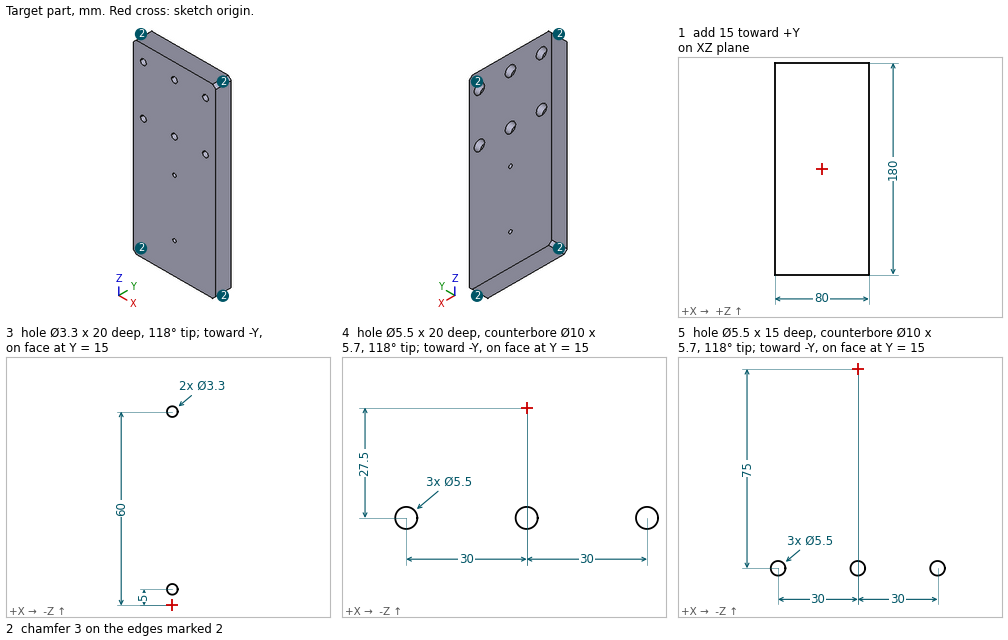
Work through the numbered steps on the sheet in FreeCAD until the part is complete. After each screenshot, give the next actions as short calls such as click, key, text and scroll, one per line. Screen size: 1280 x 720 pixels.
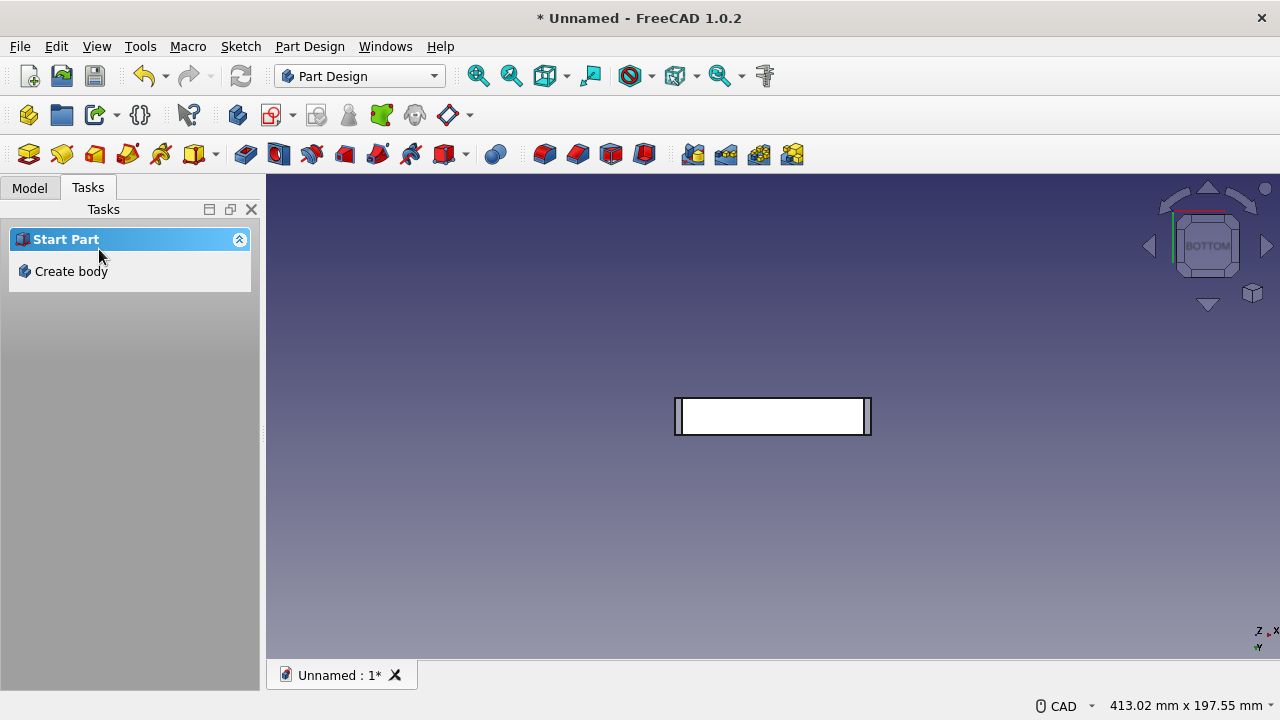
click(479, 76)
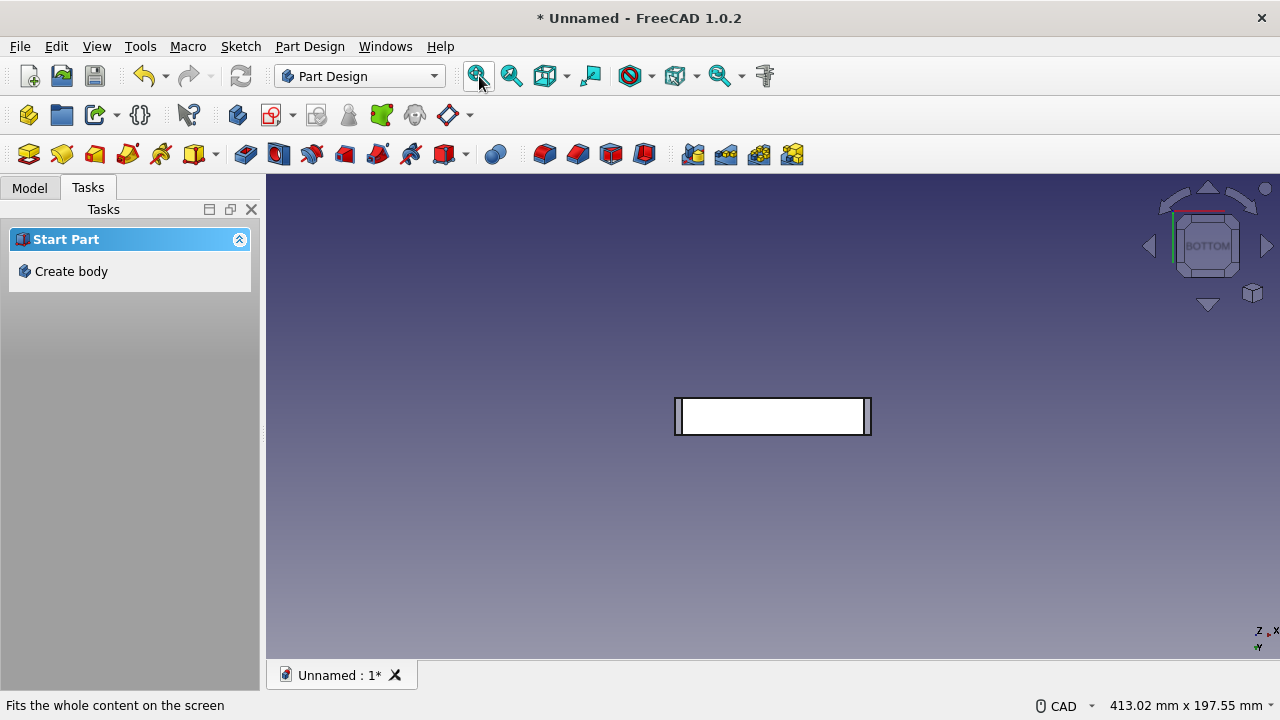
key(4)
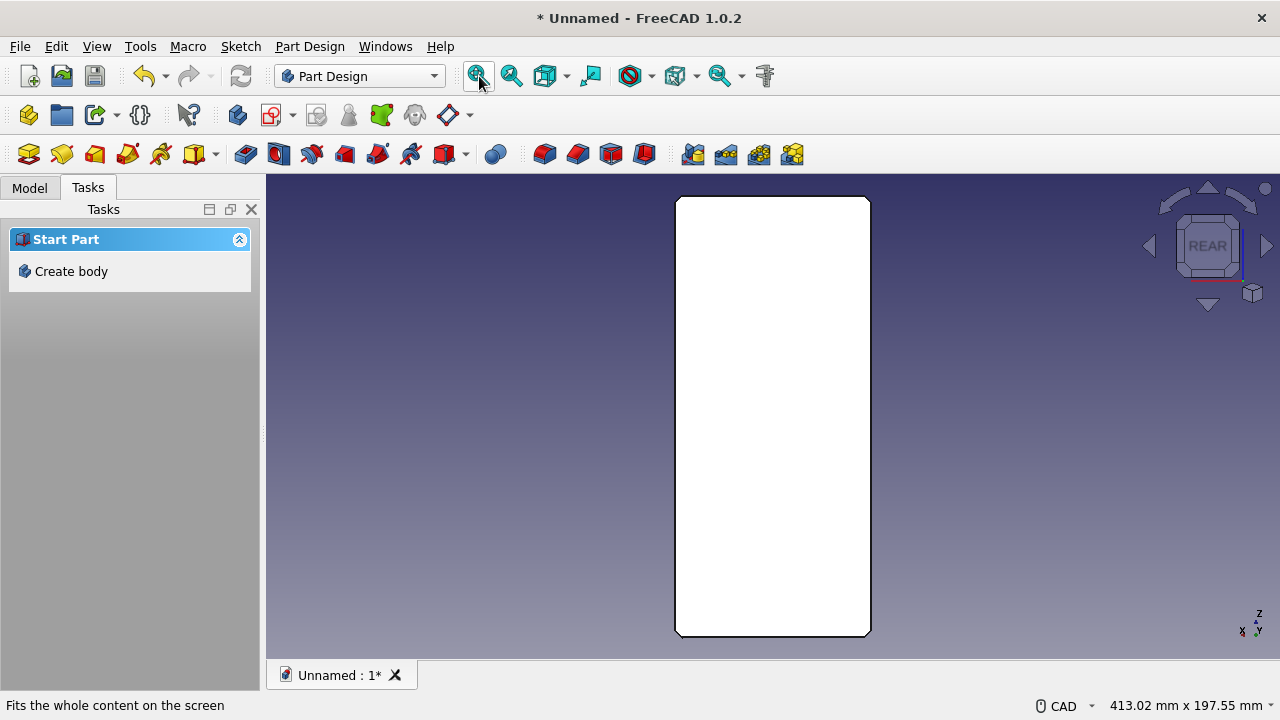
click(773, 352)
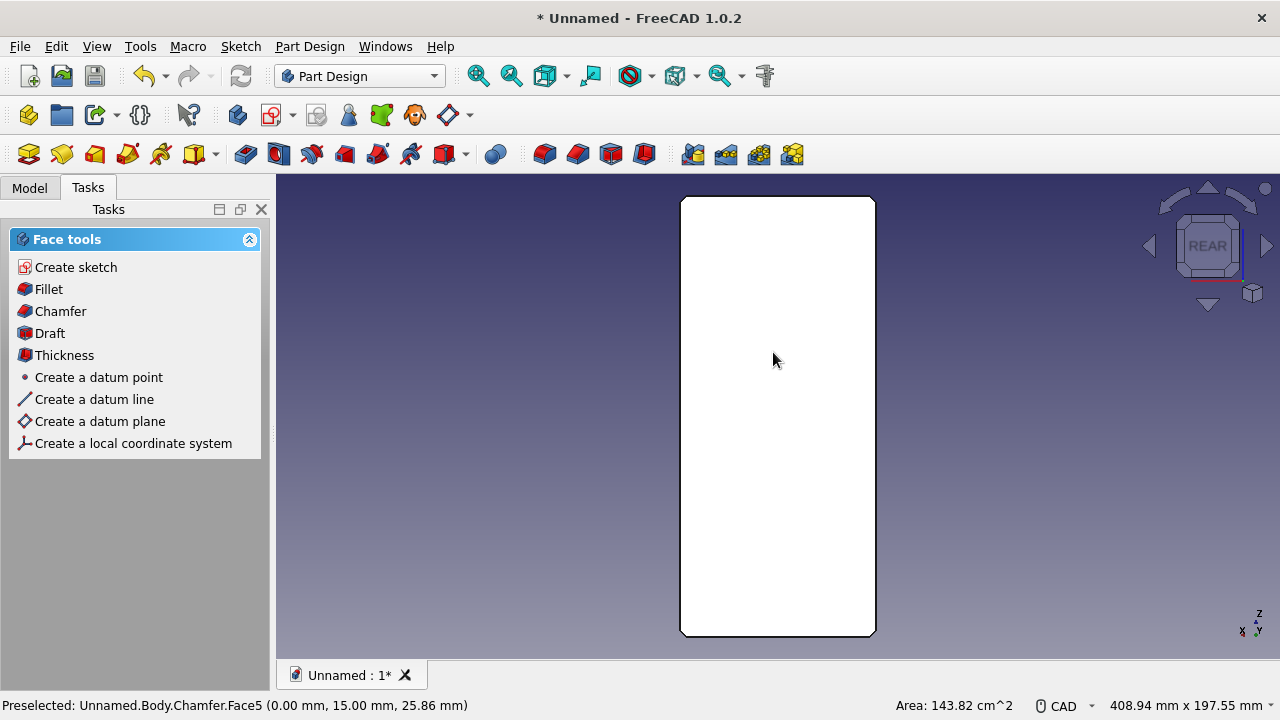
click(270, 116)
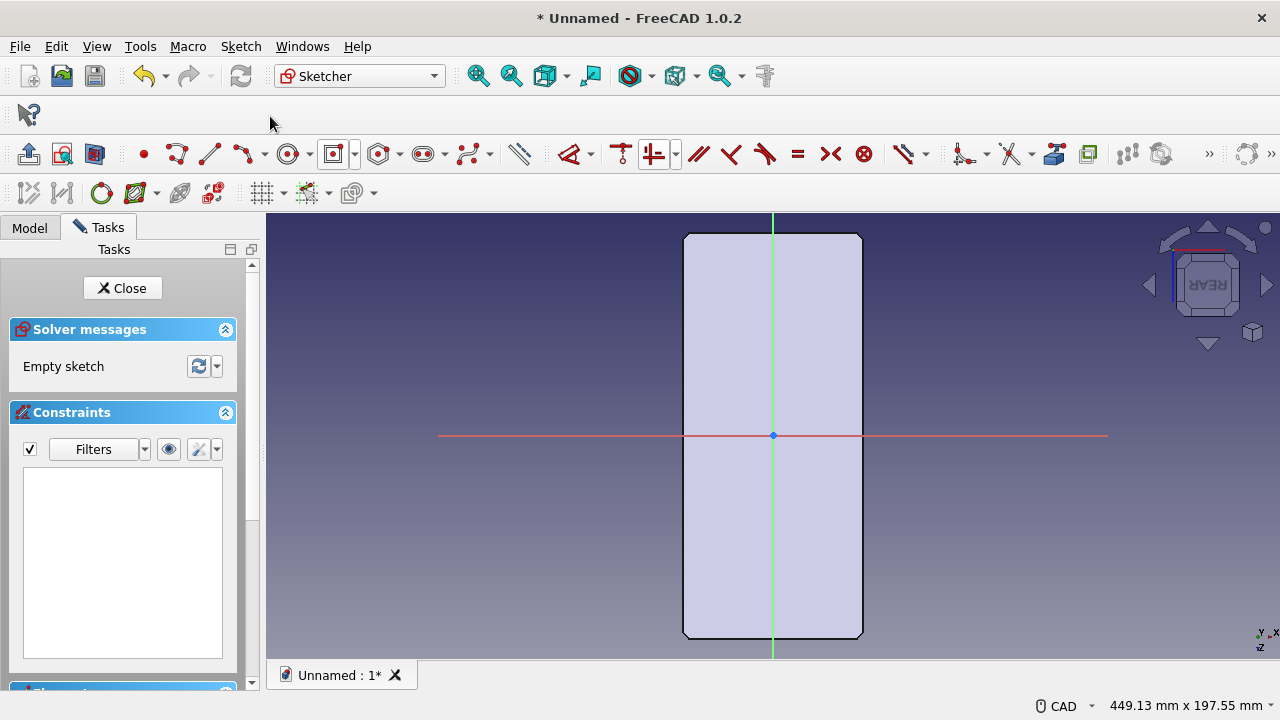
scroll(856, 282, up, 3)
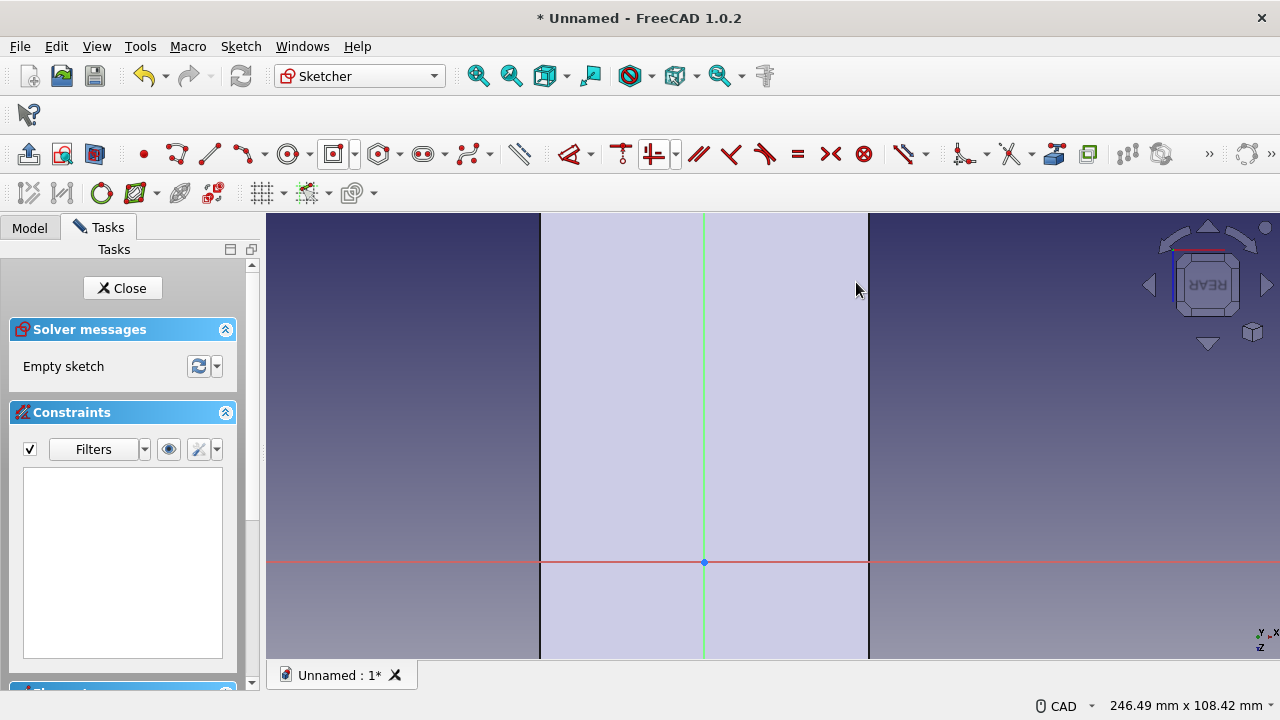
click(288, 154)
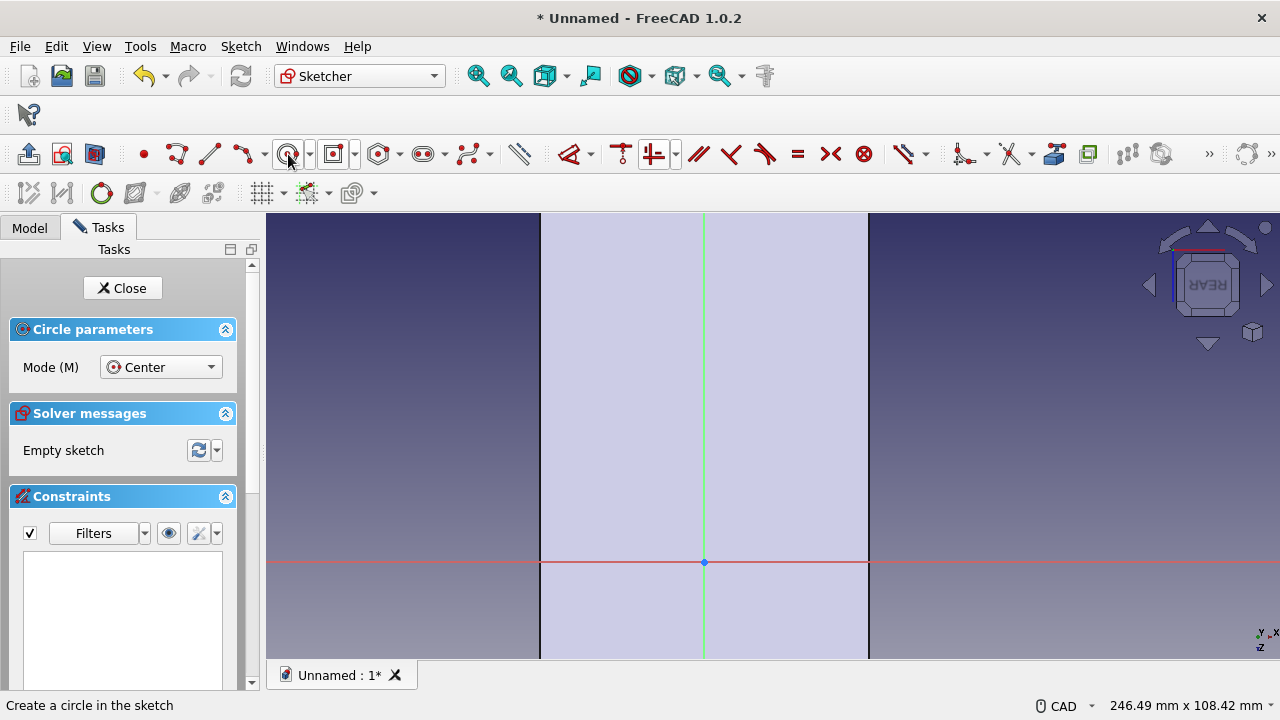
scroll(704, 316, up, 7)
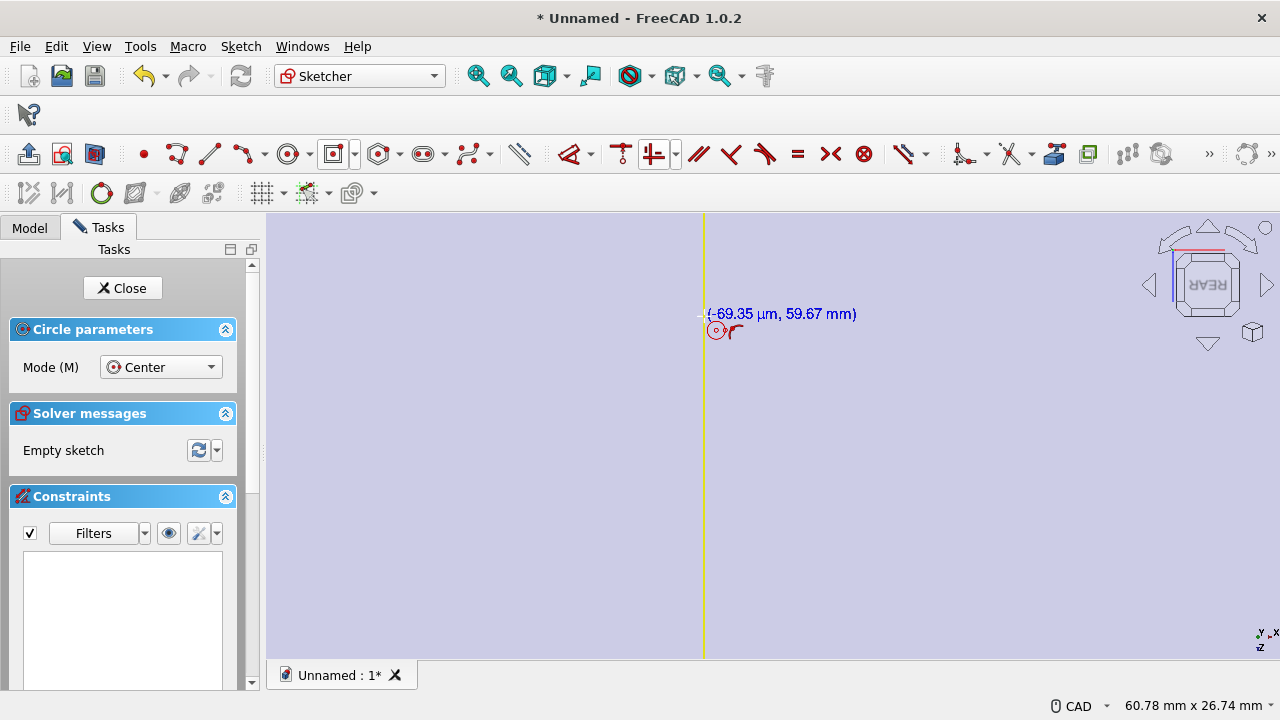
scroll(705, 317, down, 7)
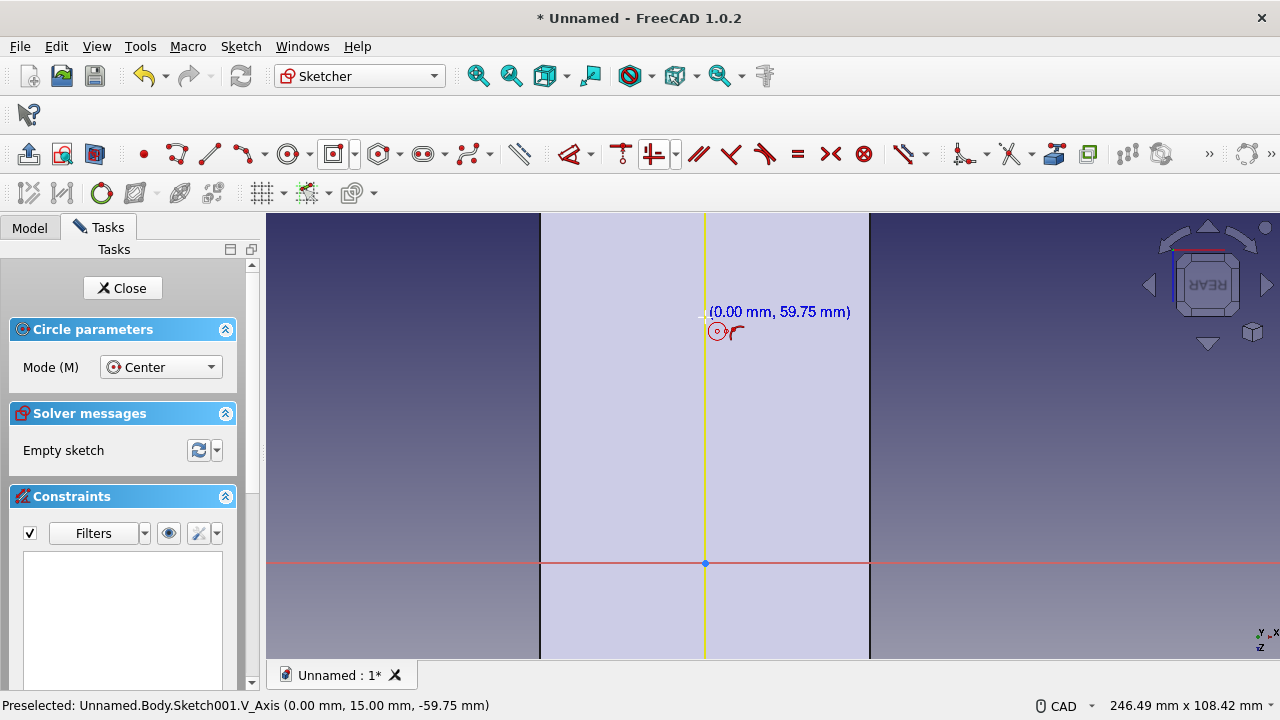
click(705, 316)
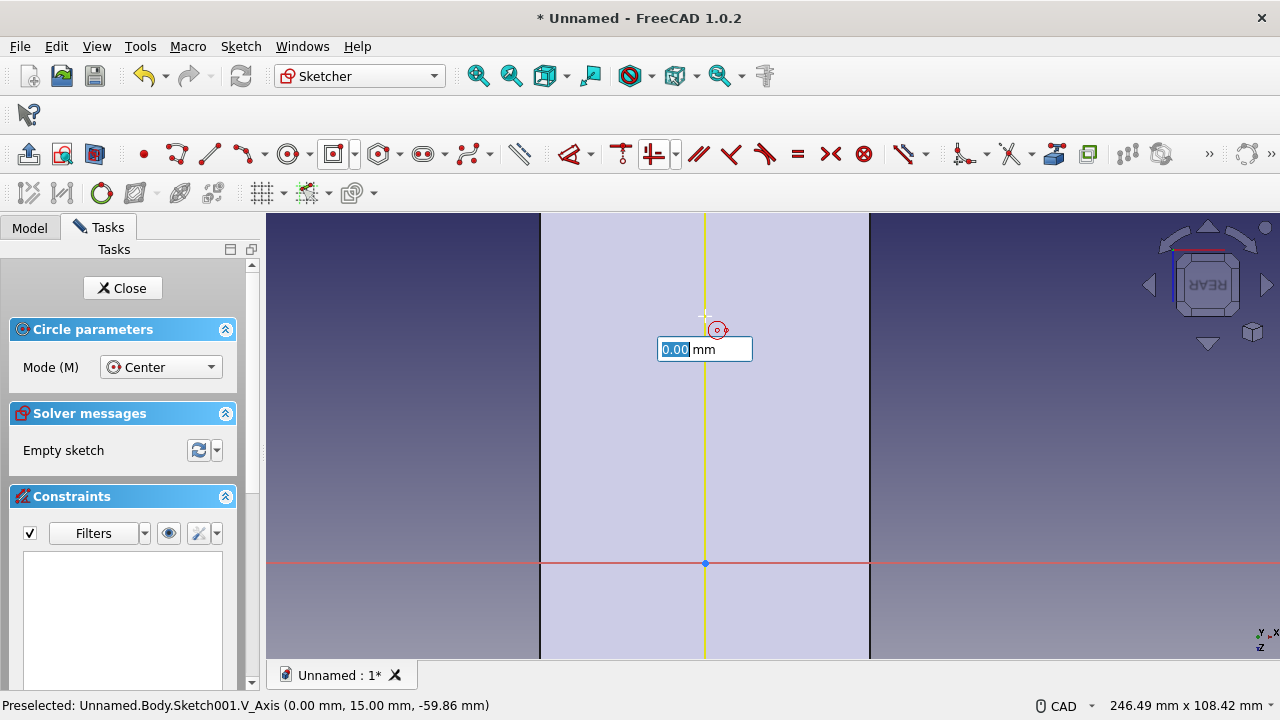
scroll(711, 314, up, 5)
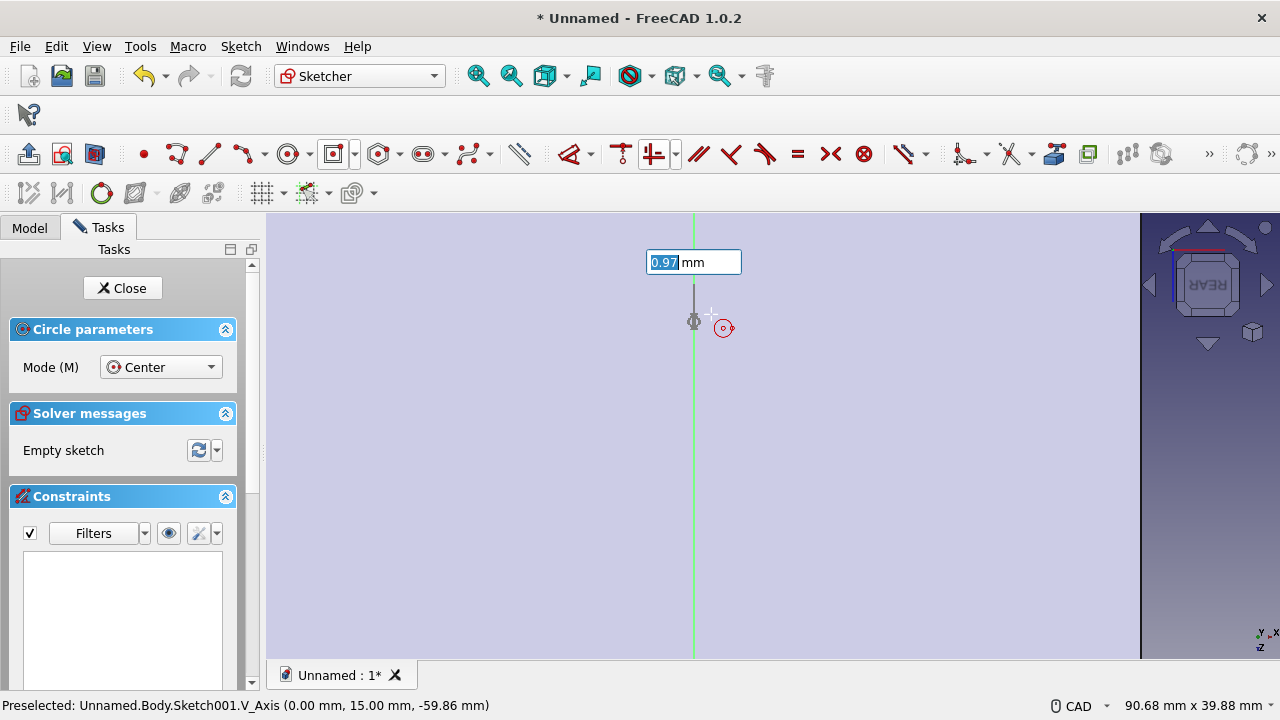
click(711, 314)